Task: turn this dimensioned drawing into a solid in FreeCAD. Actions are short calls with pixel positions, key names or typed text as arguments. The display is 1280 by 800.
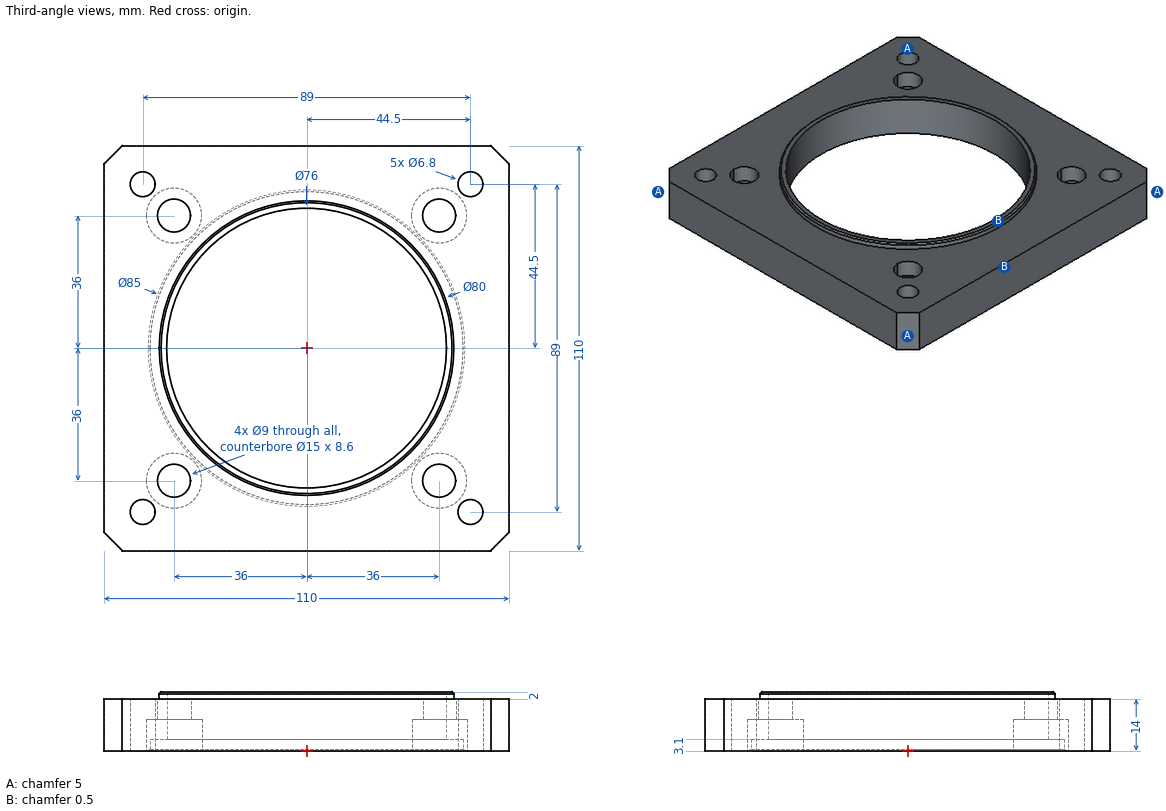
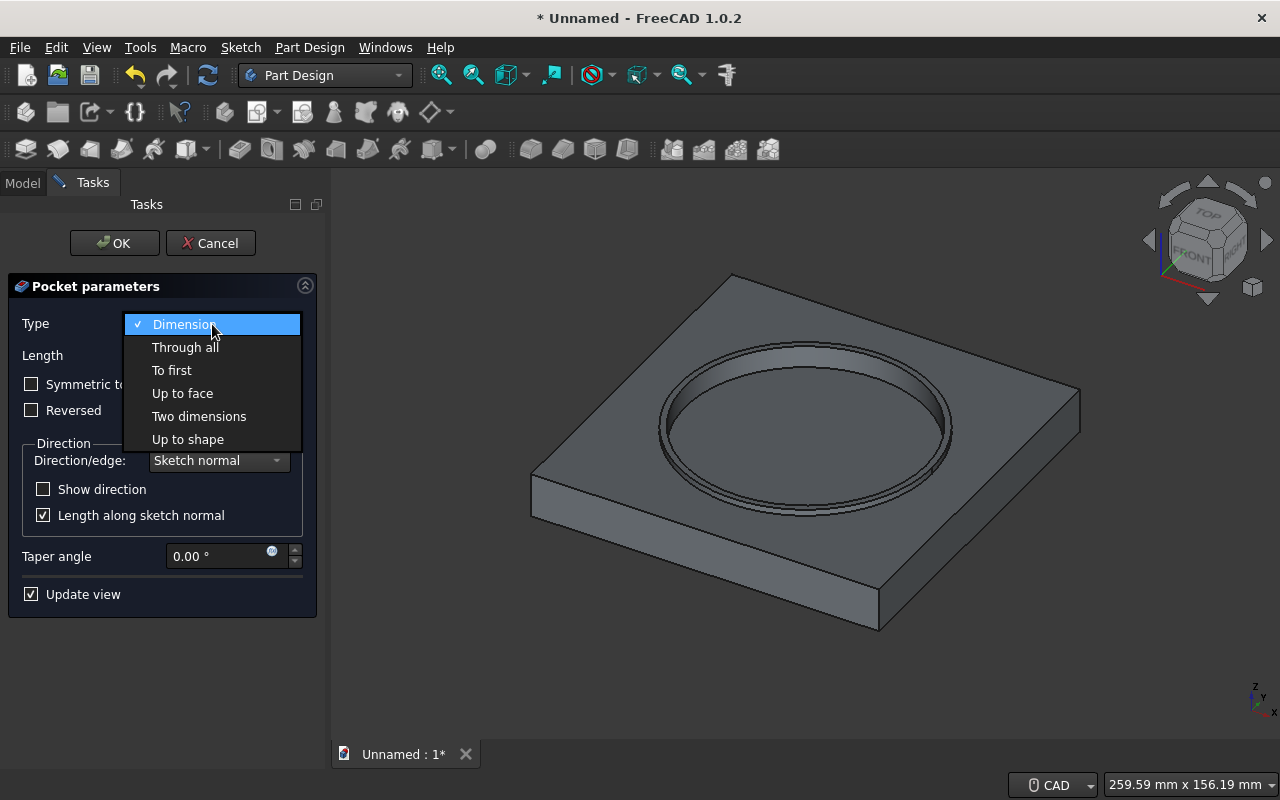
click(212, 348)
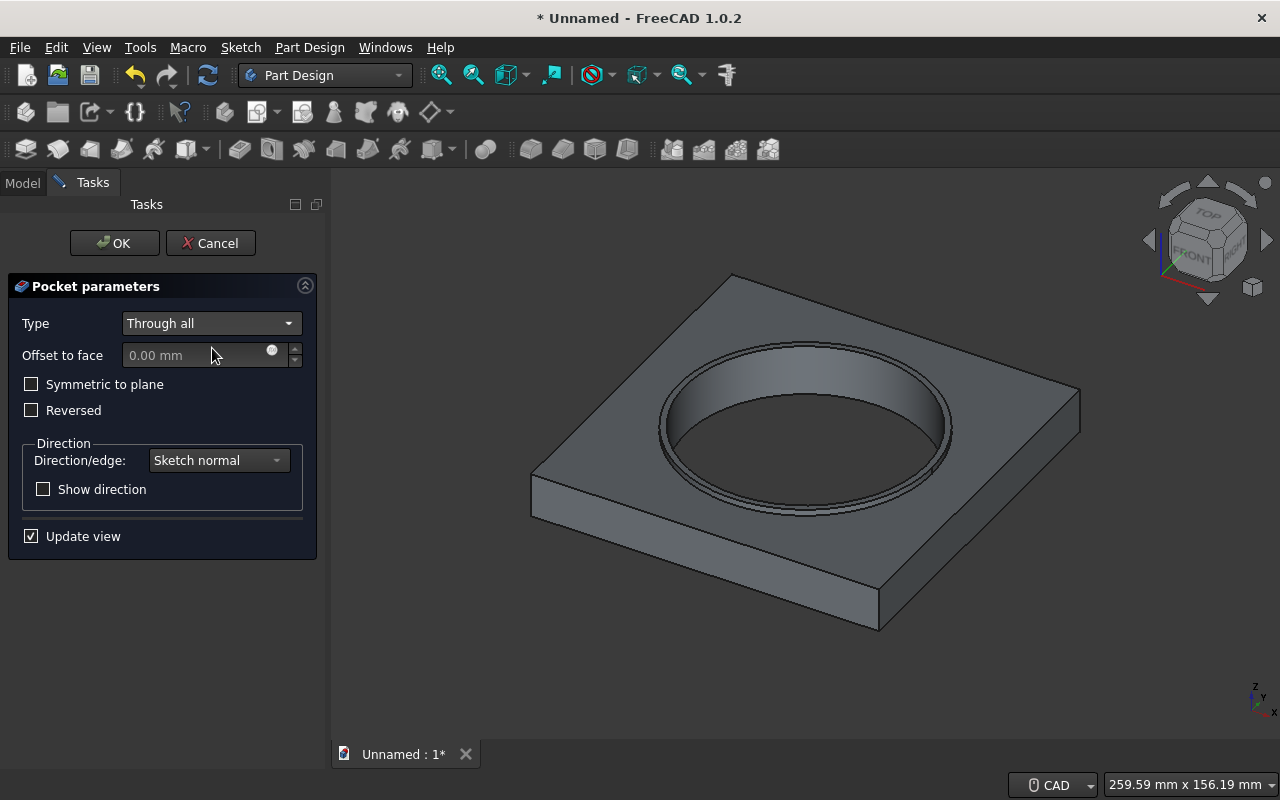
click(115, 243)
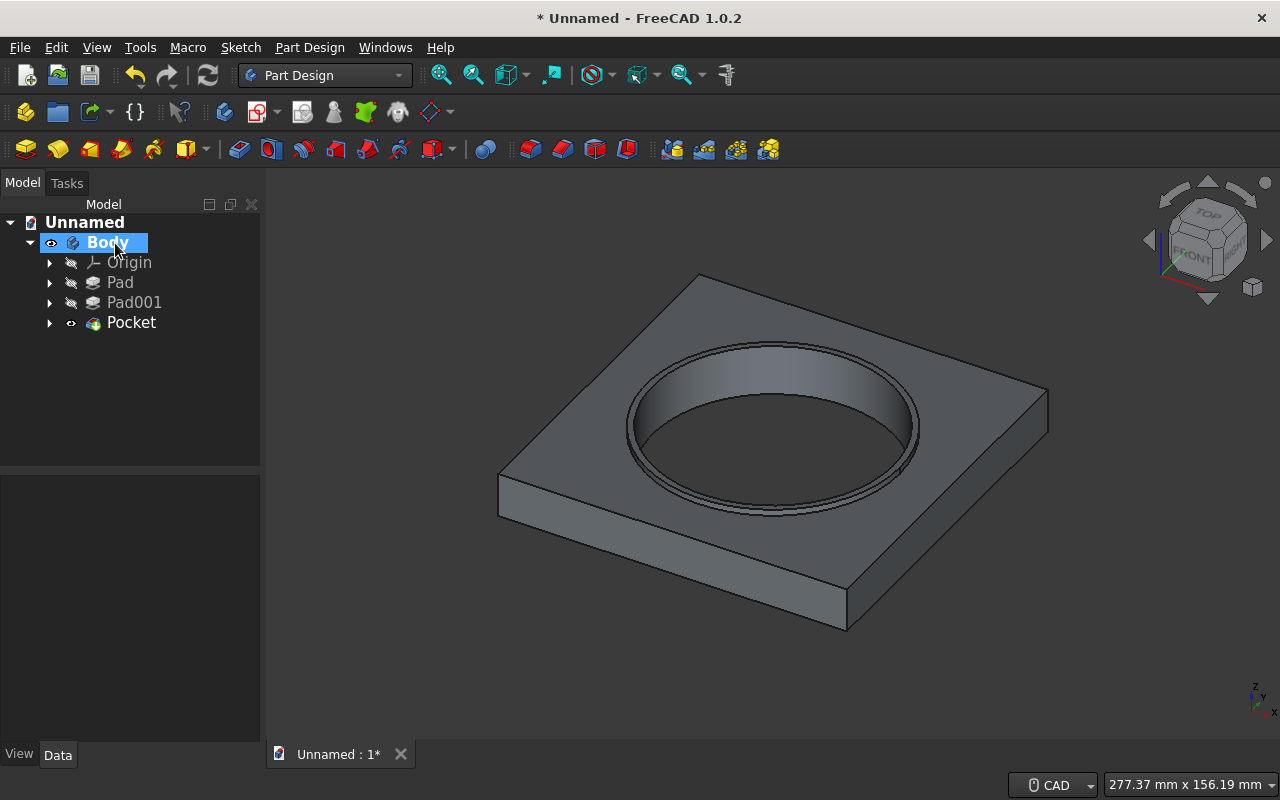
key(5)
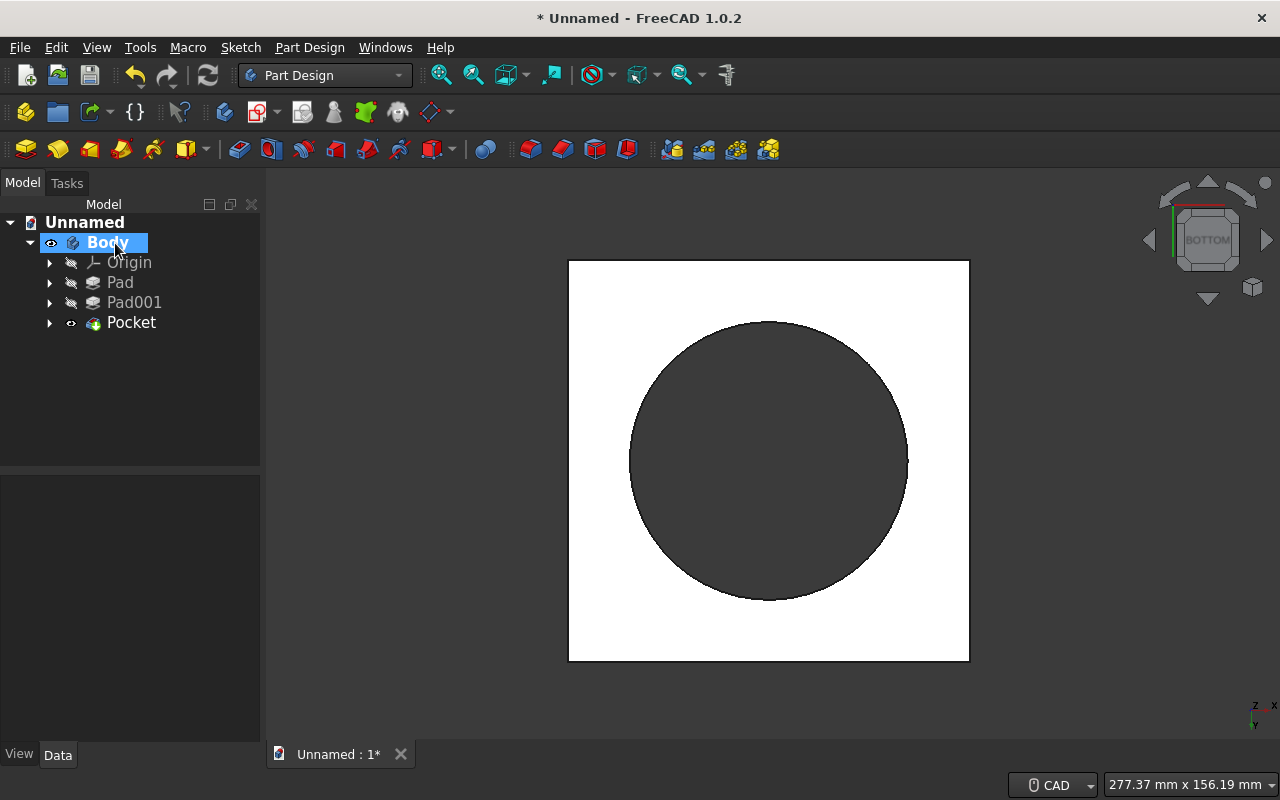
click(941, 632)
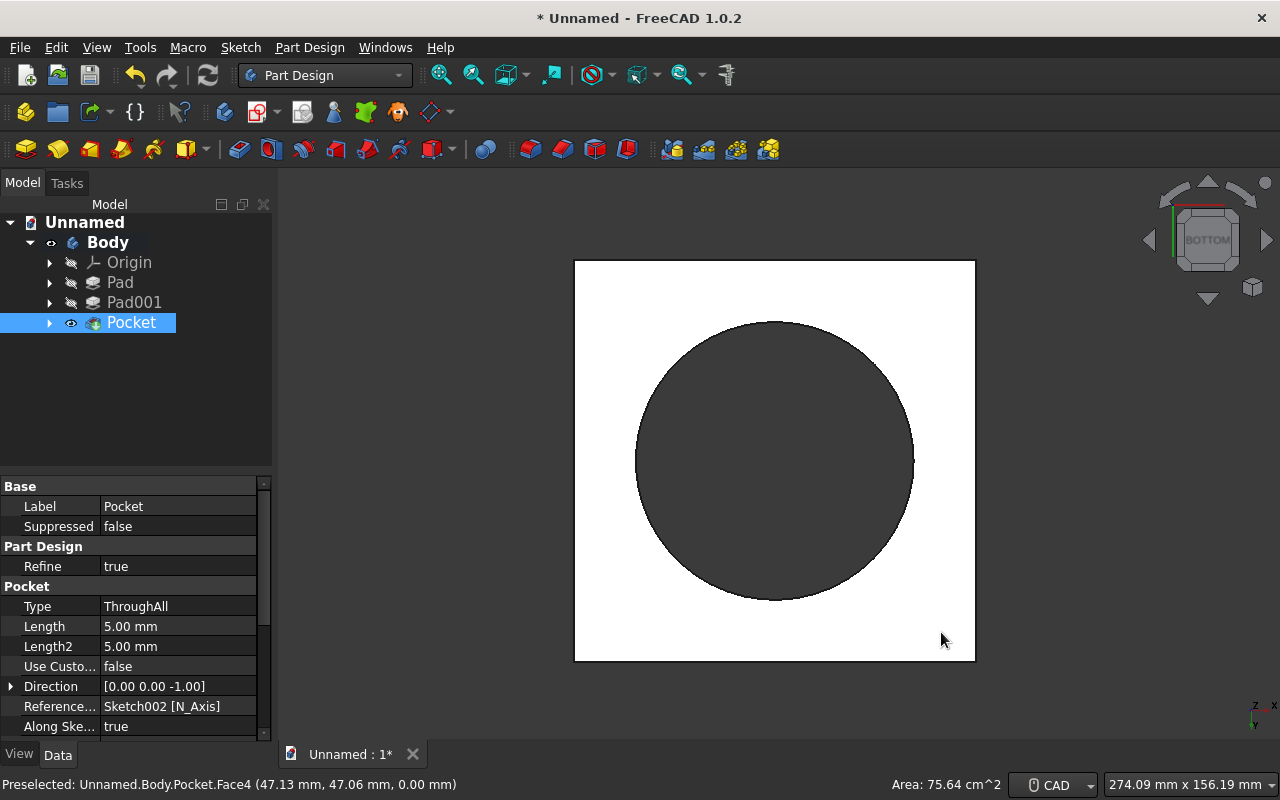
click(258, 112)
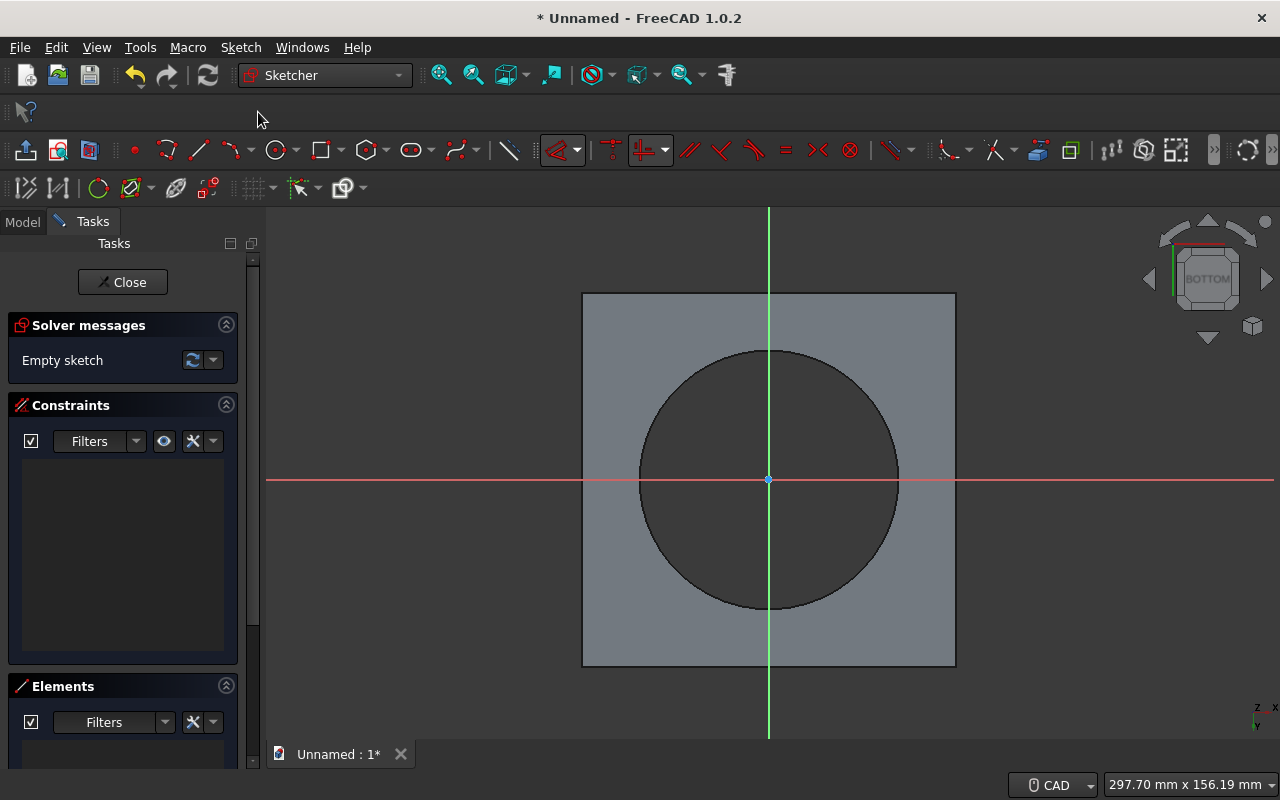
click(276, 150)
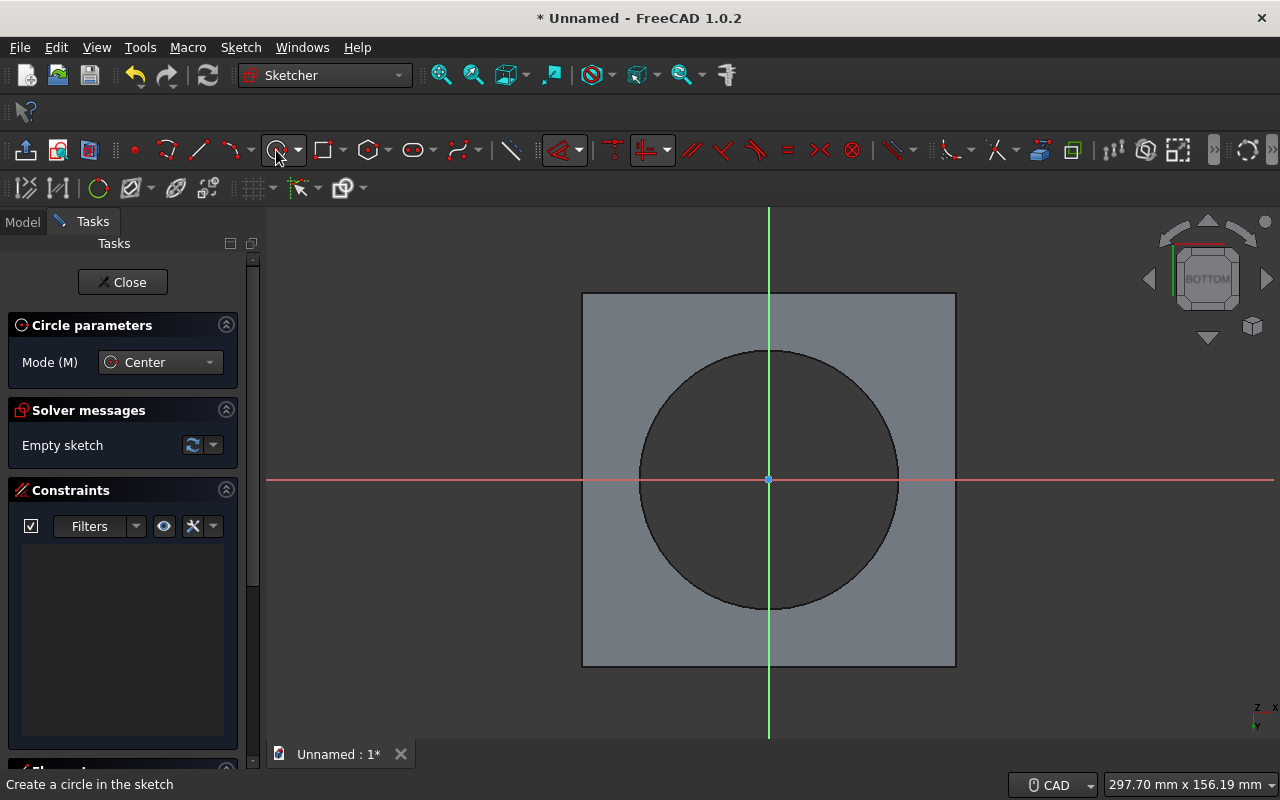
click(769, 480)
click(871, 378)
key(Escape)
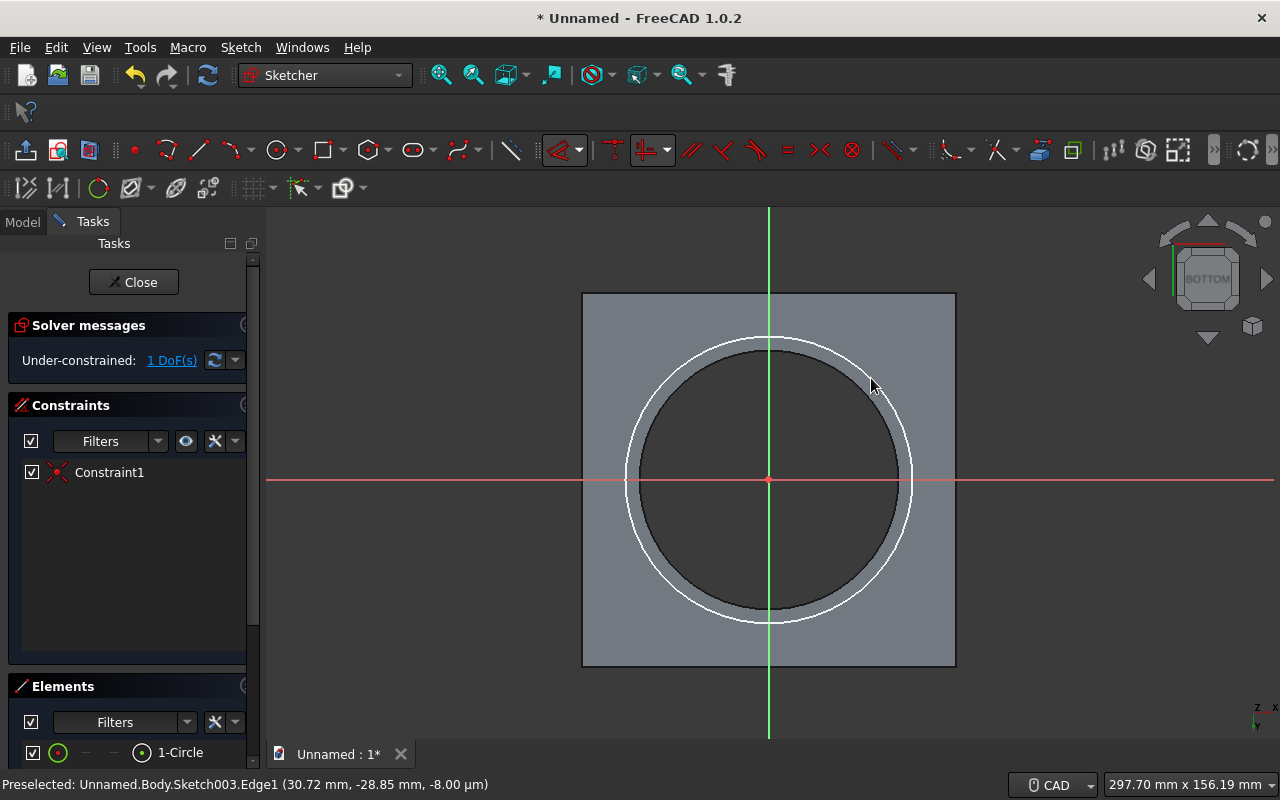
click(870, 378)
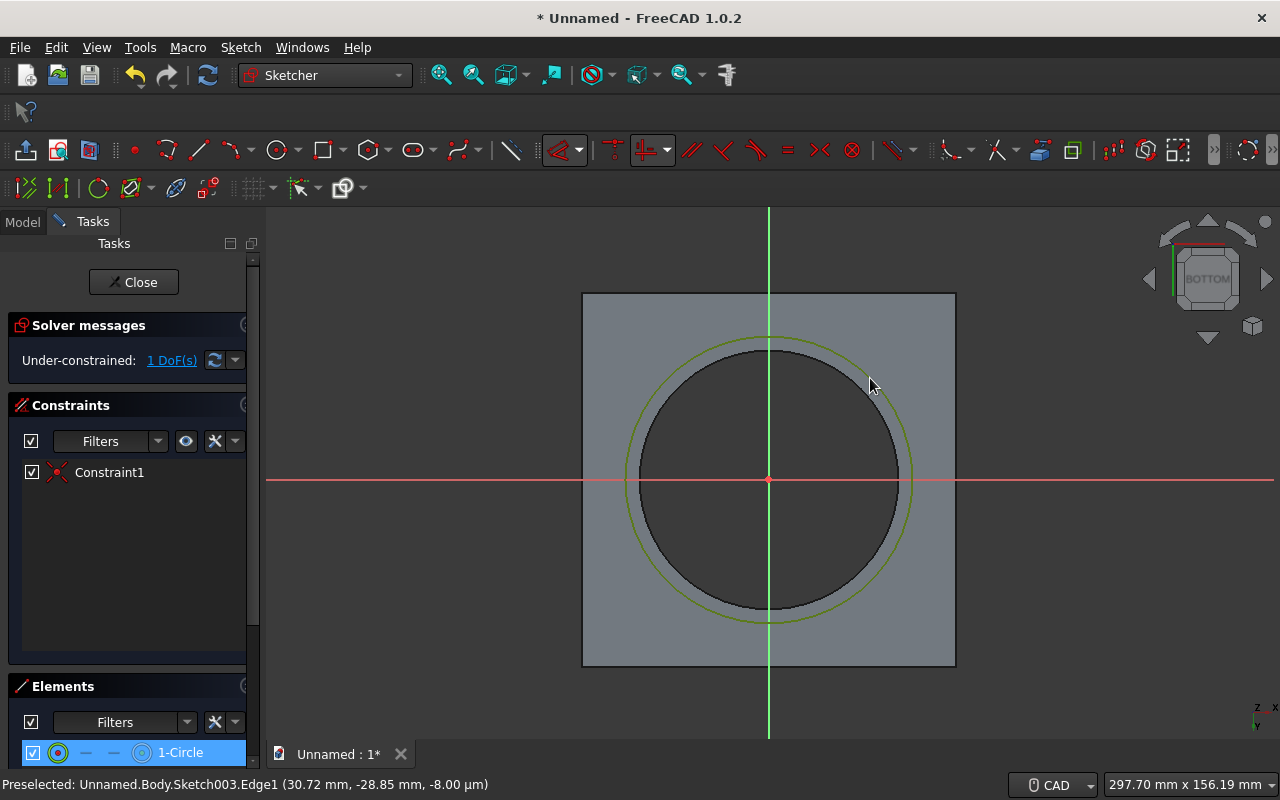
click(582, 150)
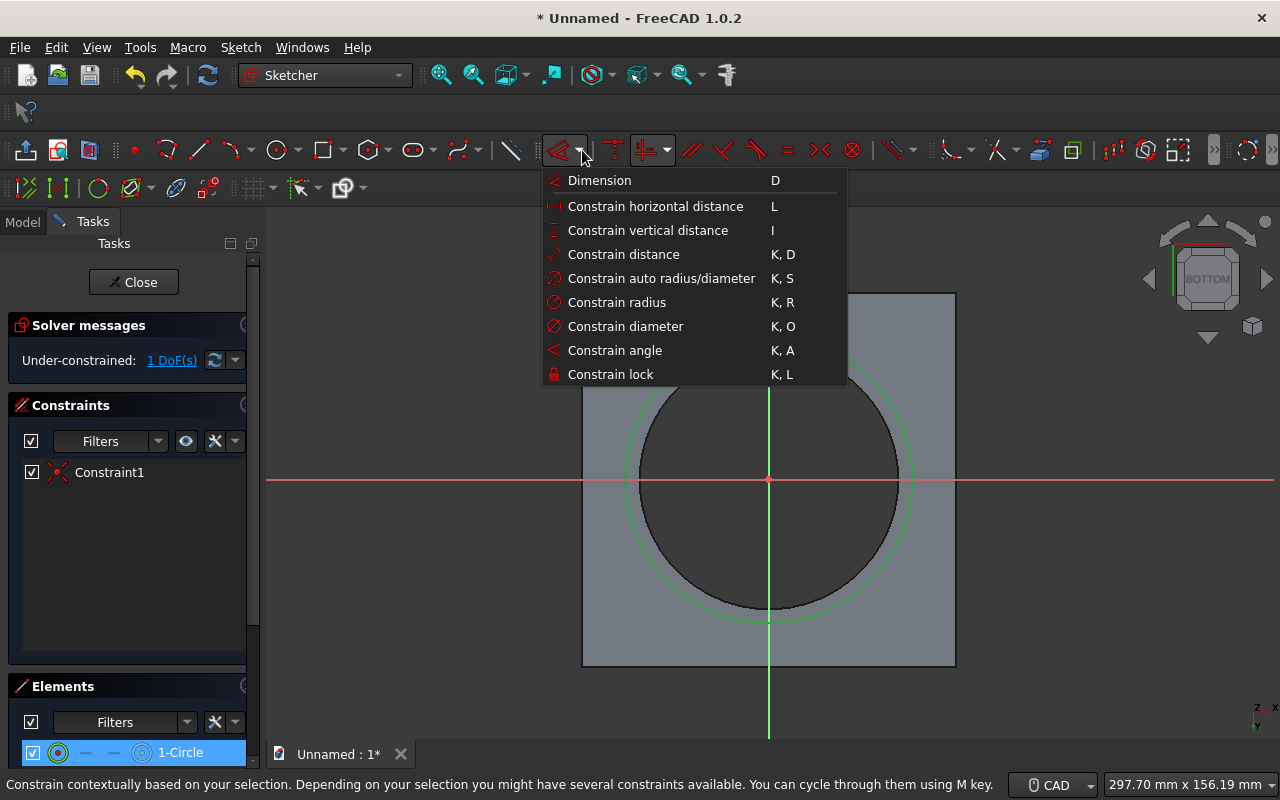
click(695, 326)